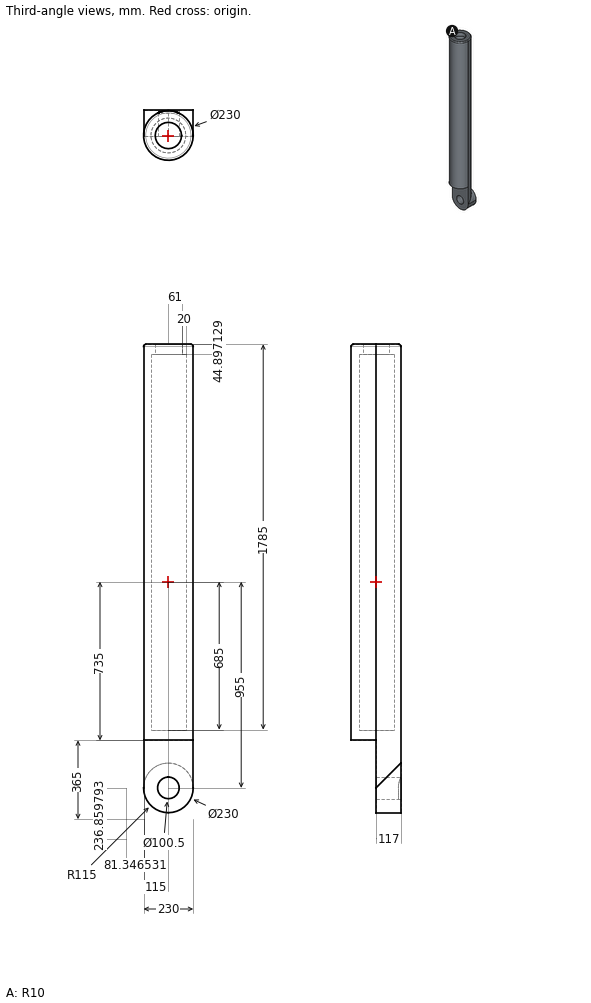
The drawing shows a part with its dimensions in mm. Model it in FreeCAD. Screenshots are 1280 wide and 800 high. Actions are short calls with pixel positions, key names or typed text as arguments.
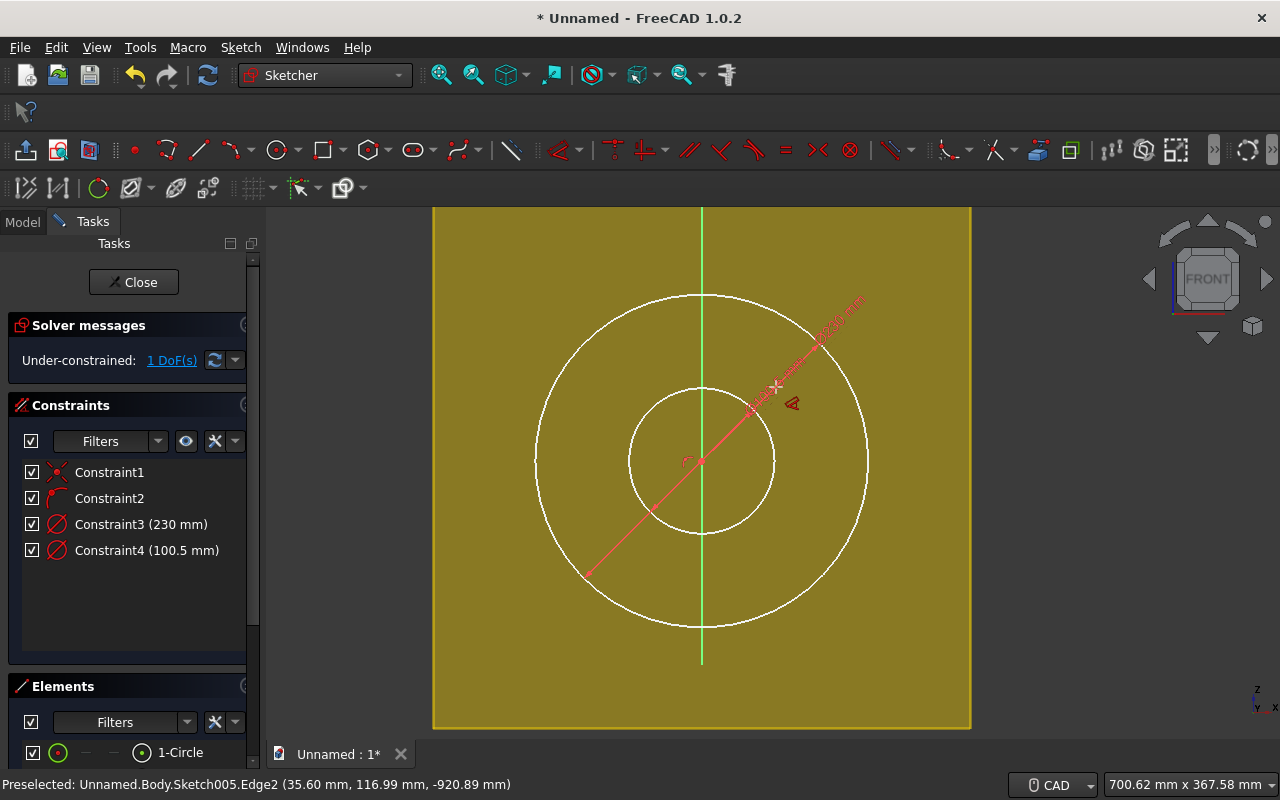
click(702, 461)
click(736, 348)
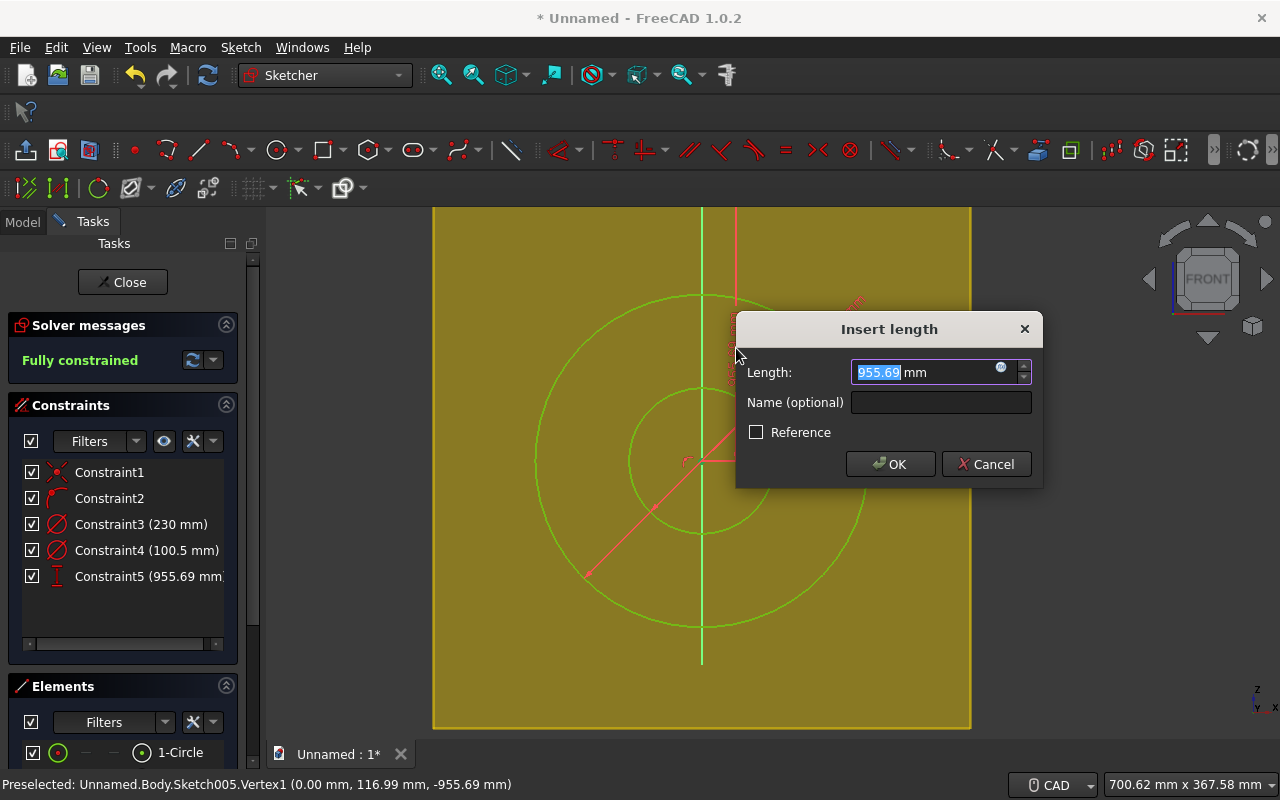
text(955)
key(Return)
key(Escape)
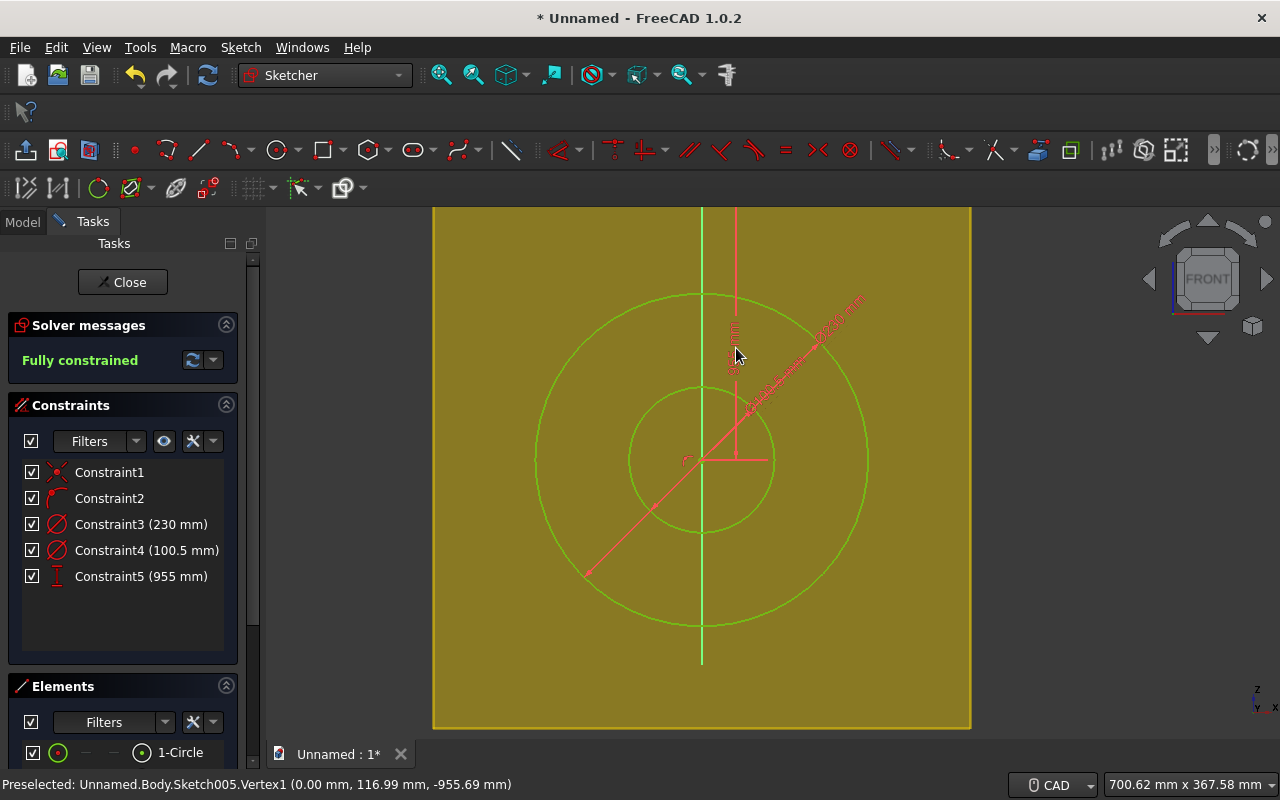
click(123, 282)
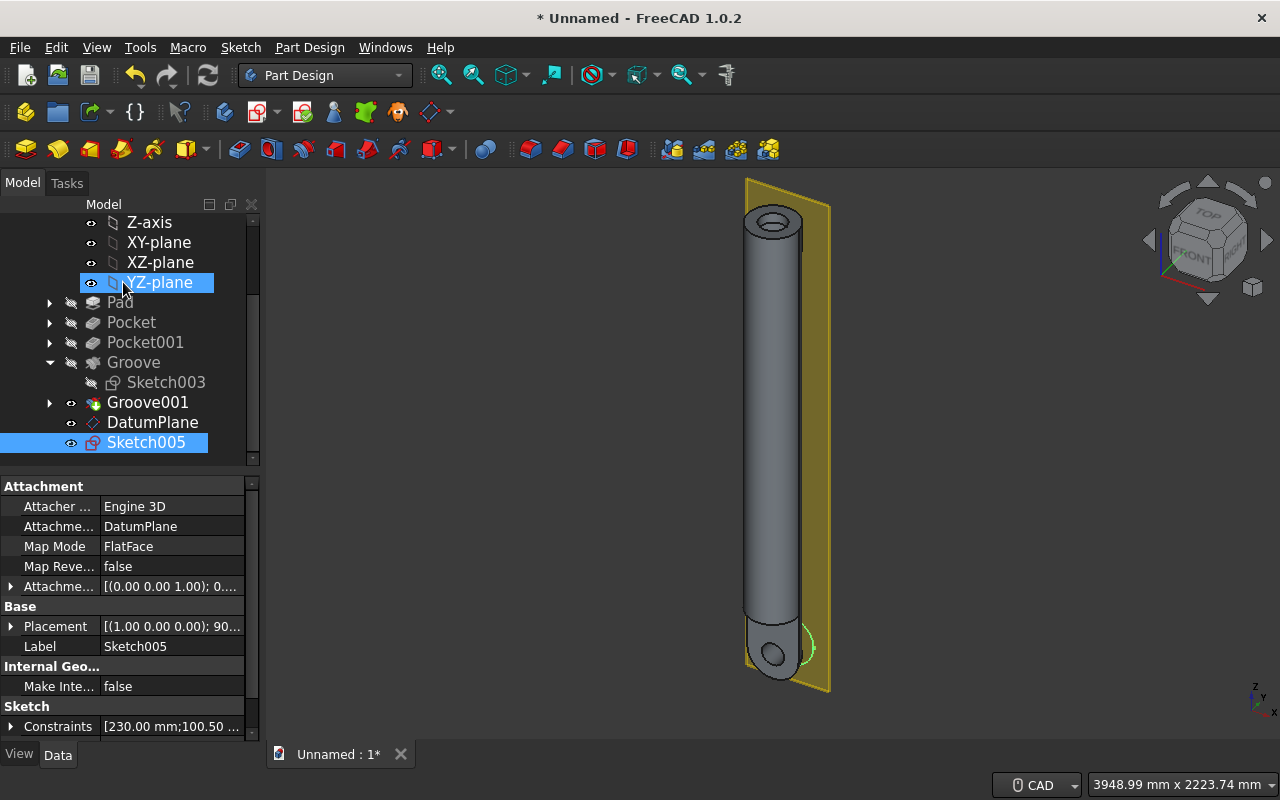
click(26, 150)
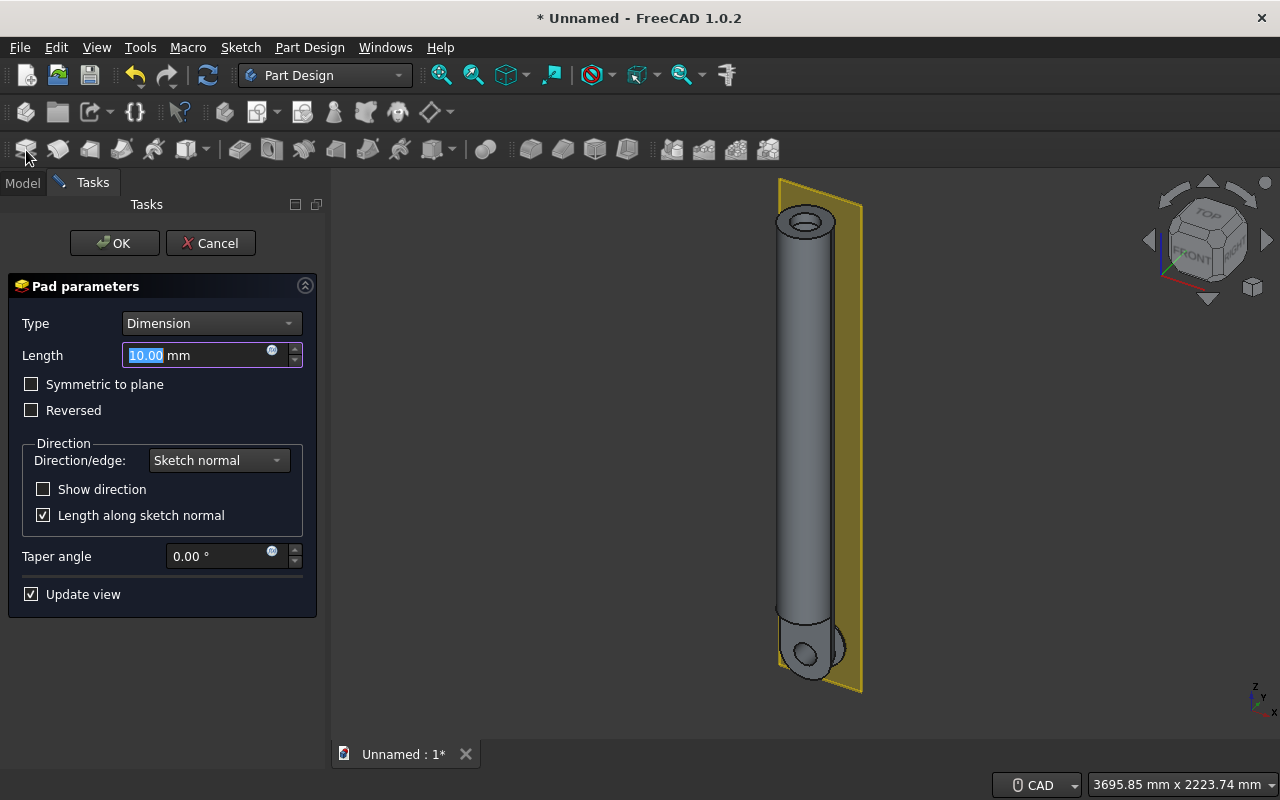
text(117)
key(Tab)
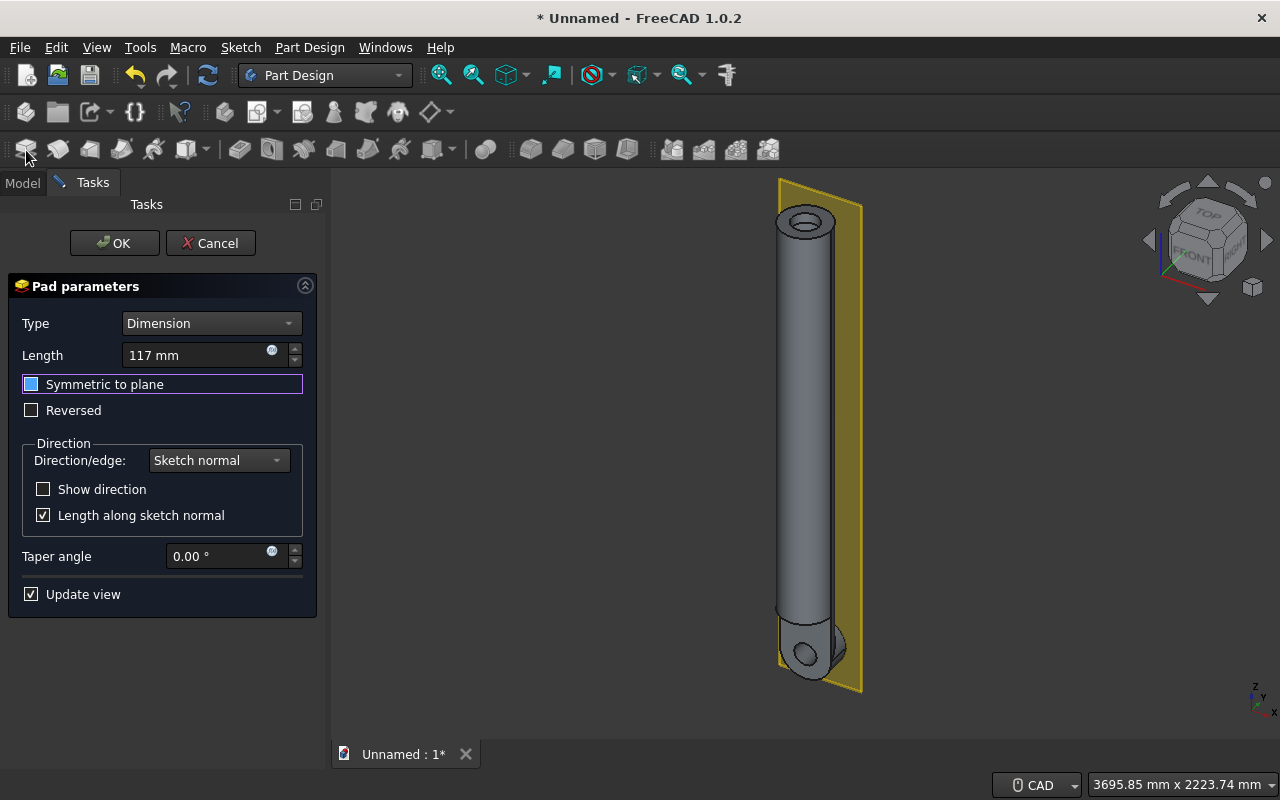
click(115, 243)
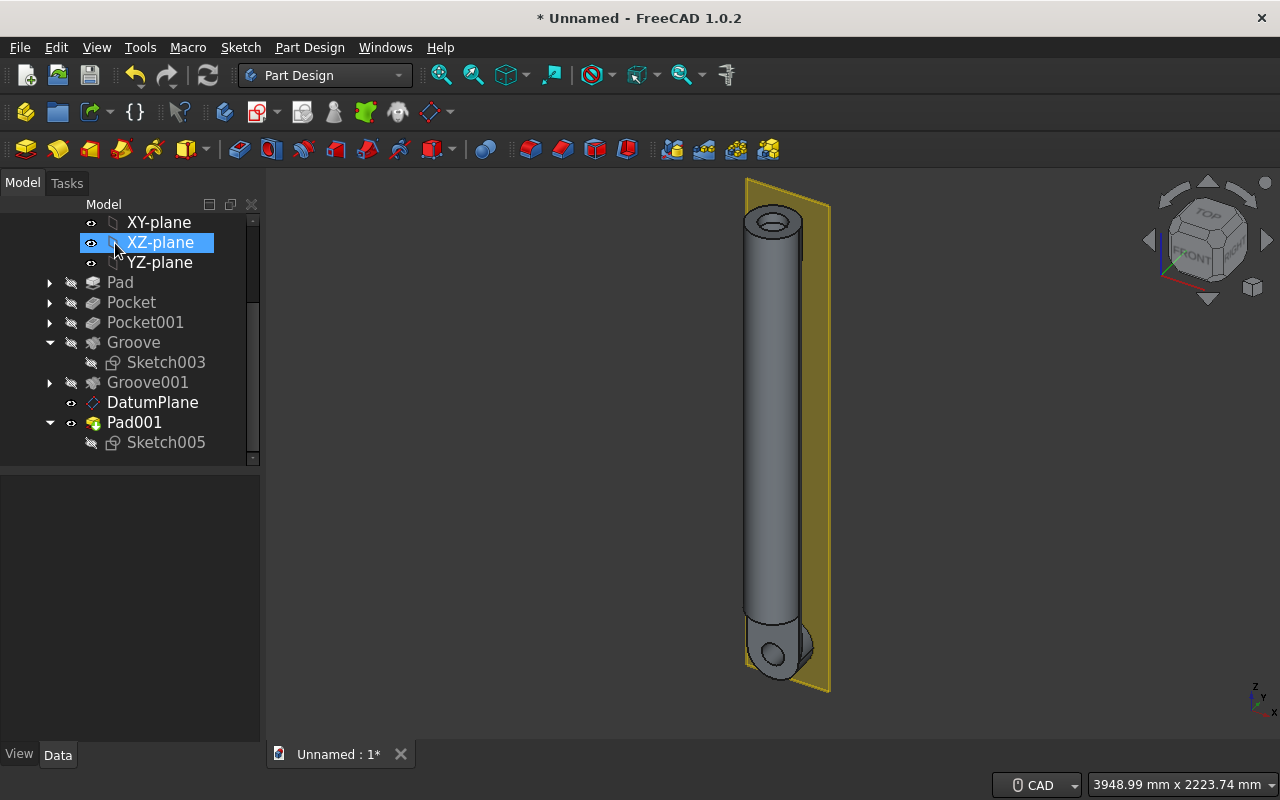
click(116, 403)
key(space)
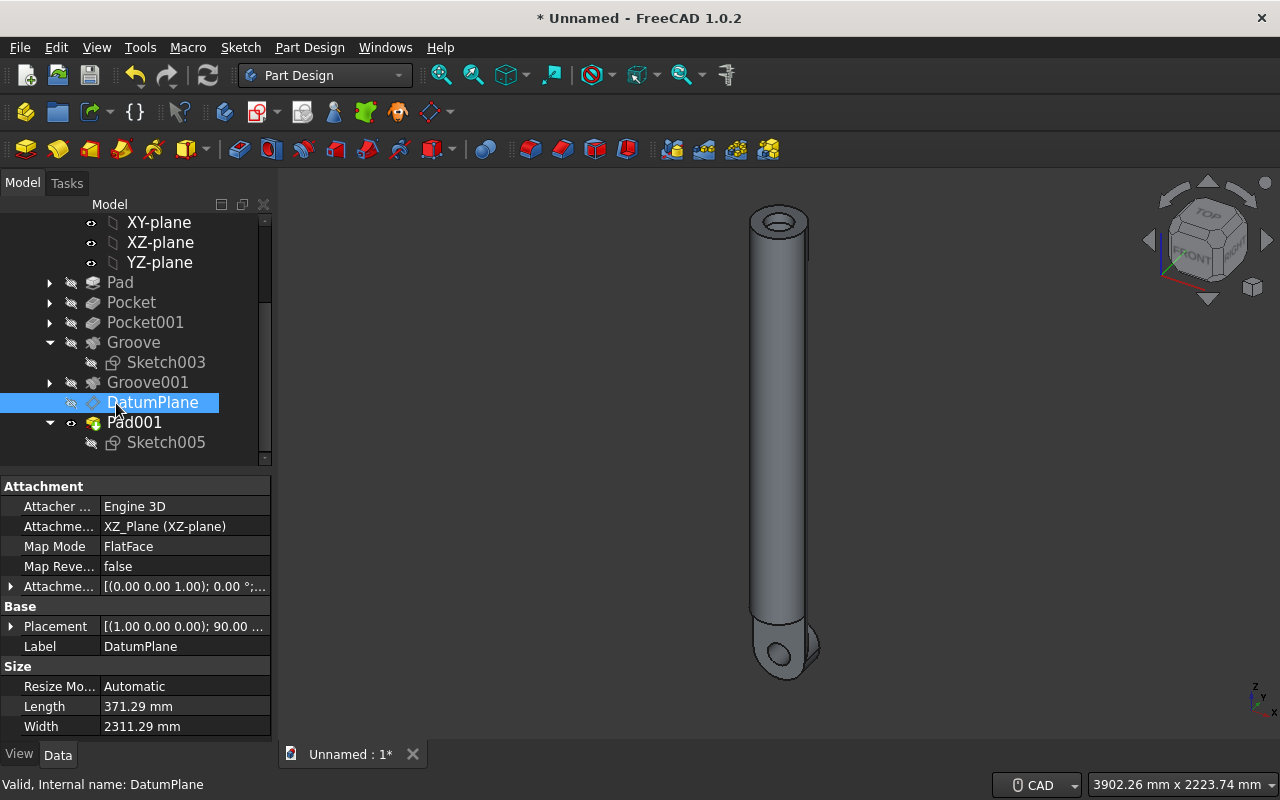
click(750, 223)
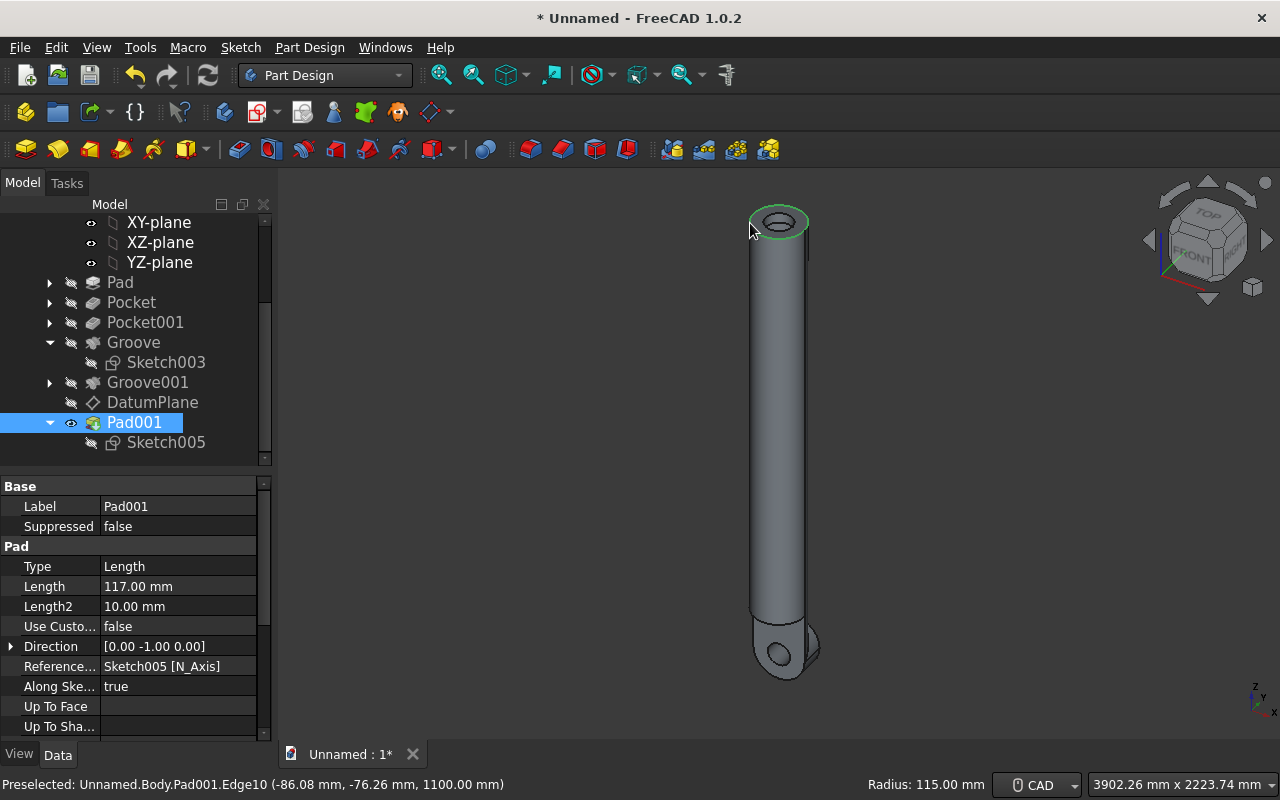
click(532, 150)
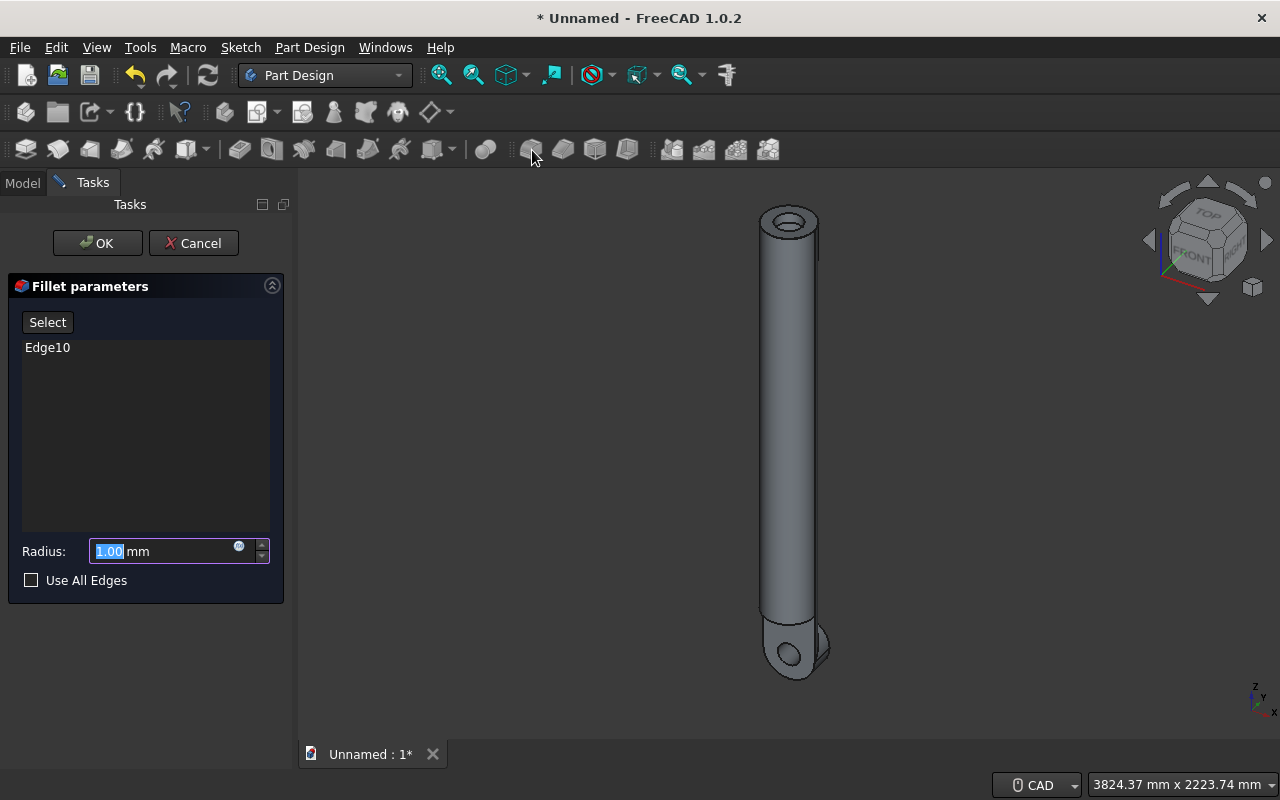
text(10)
key(Tab)